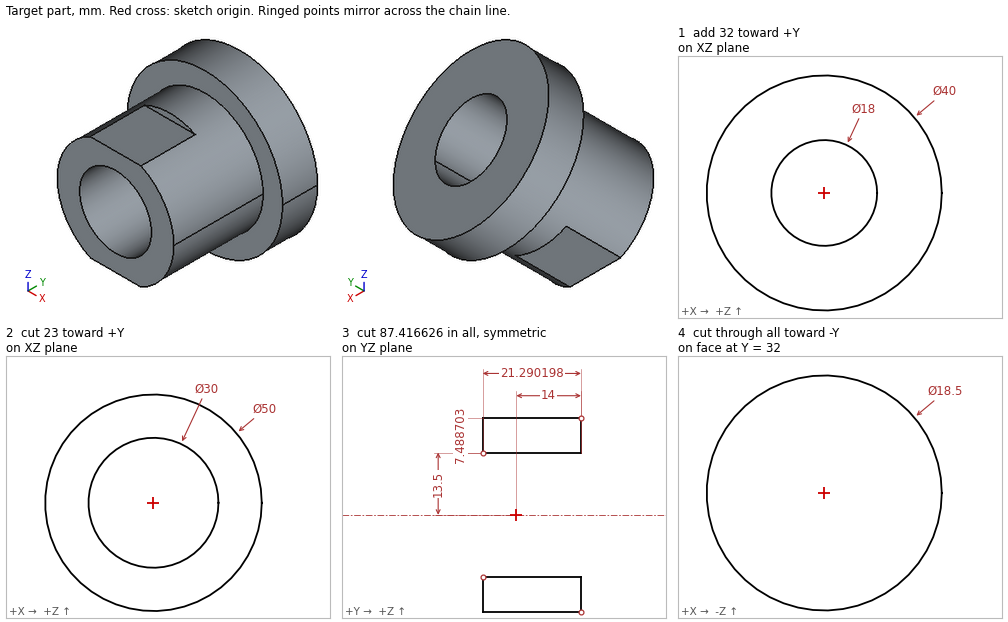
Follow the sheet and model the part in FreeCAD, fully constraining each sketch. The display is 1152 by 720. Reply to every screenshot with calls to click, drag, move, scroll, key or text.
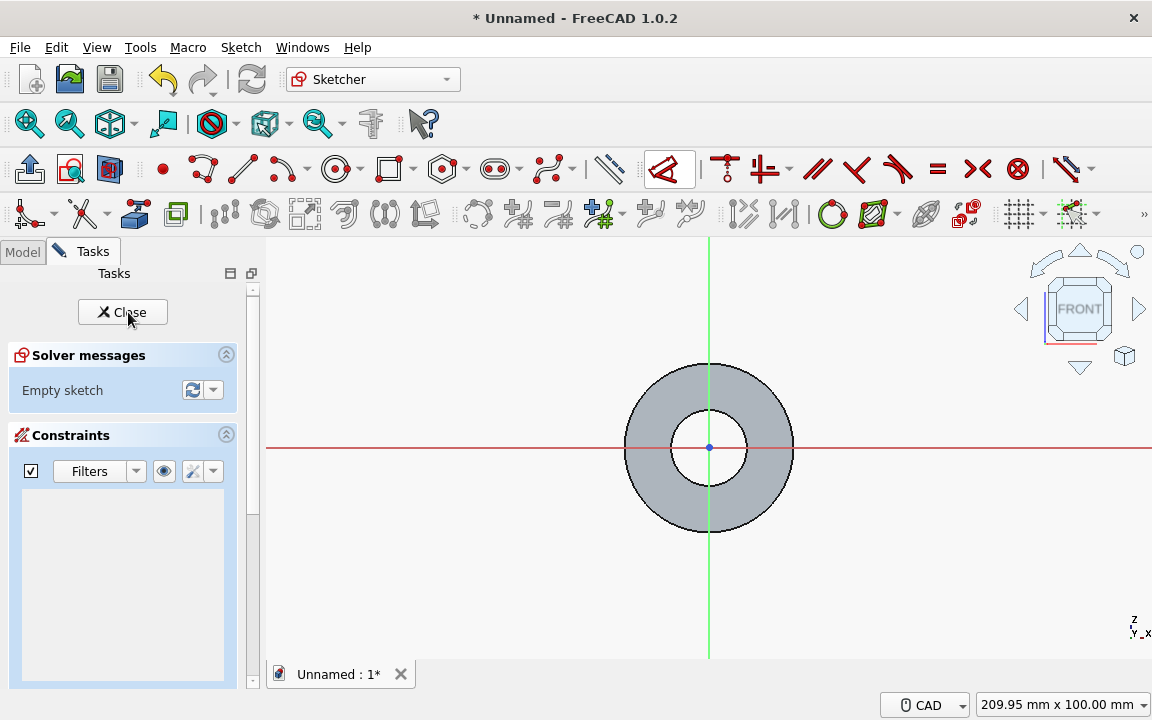
click(336, 170)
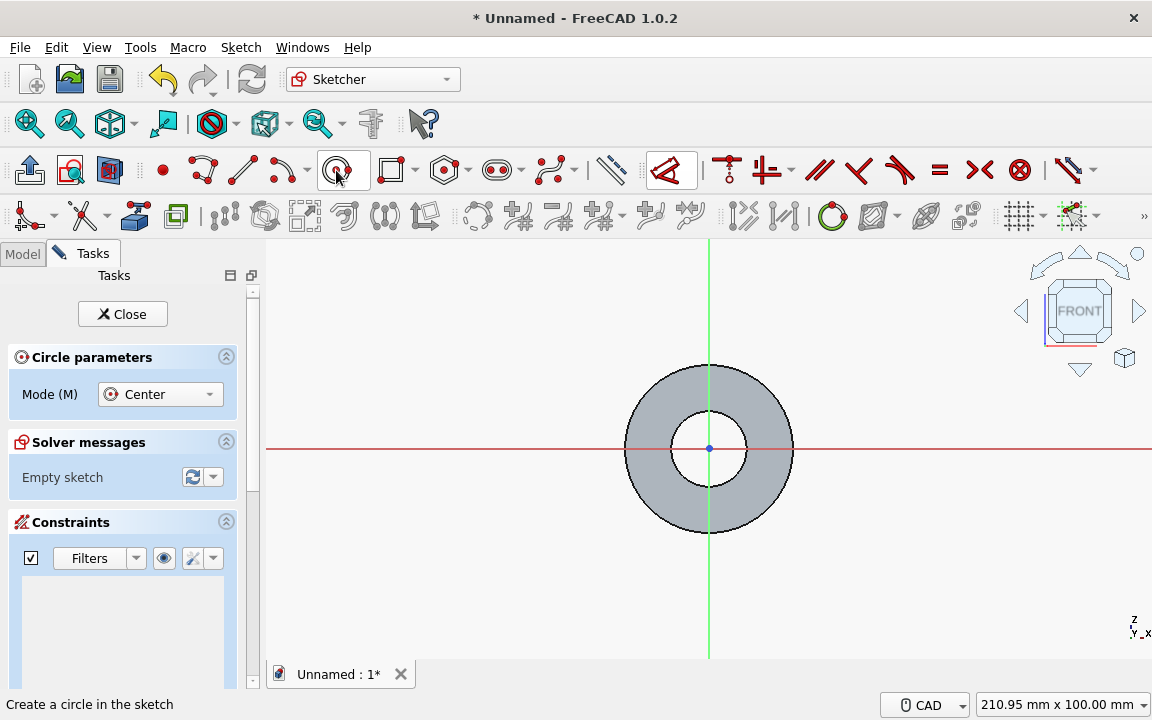
click(709, 449)
click(783, 375)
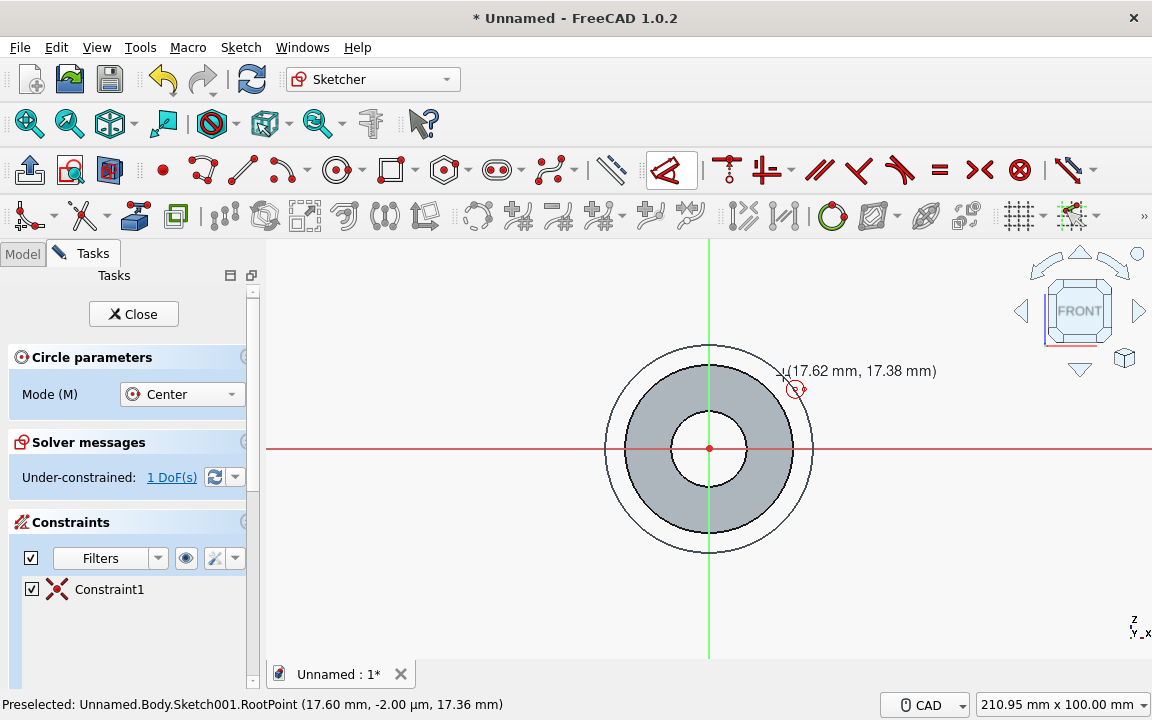
click(709, 449)
click(754, 404)
key(Escape)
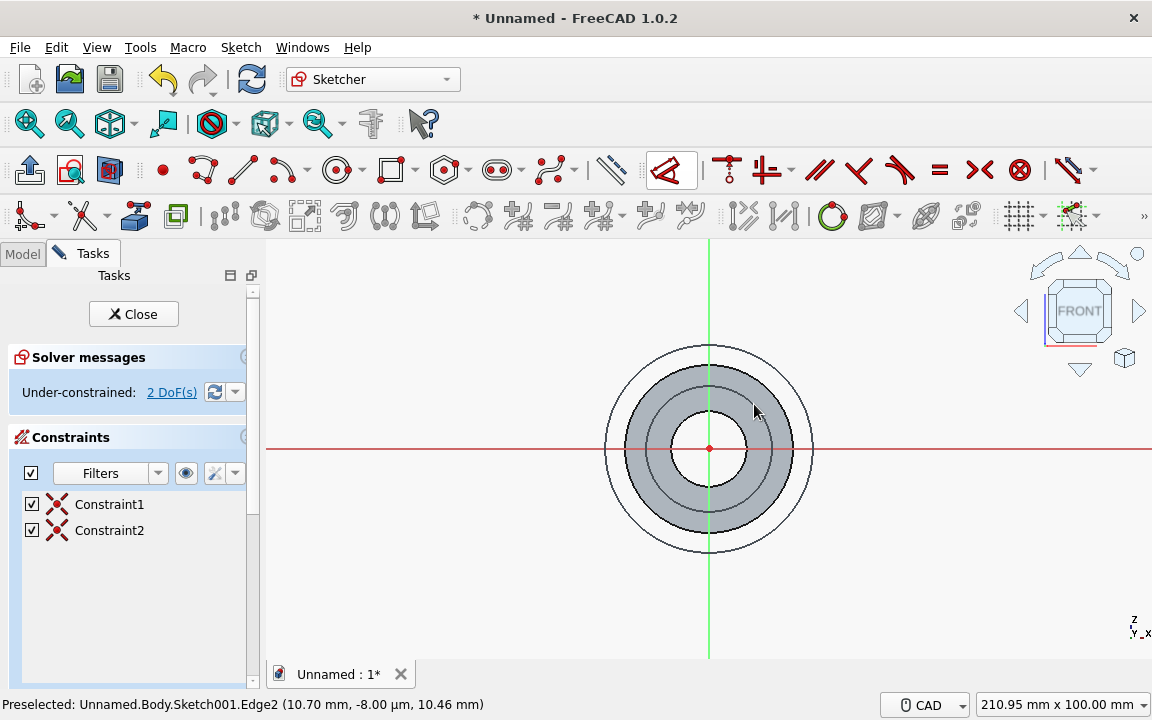
click(782, 375)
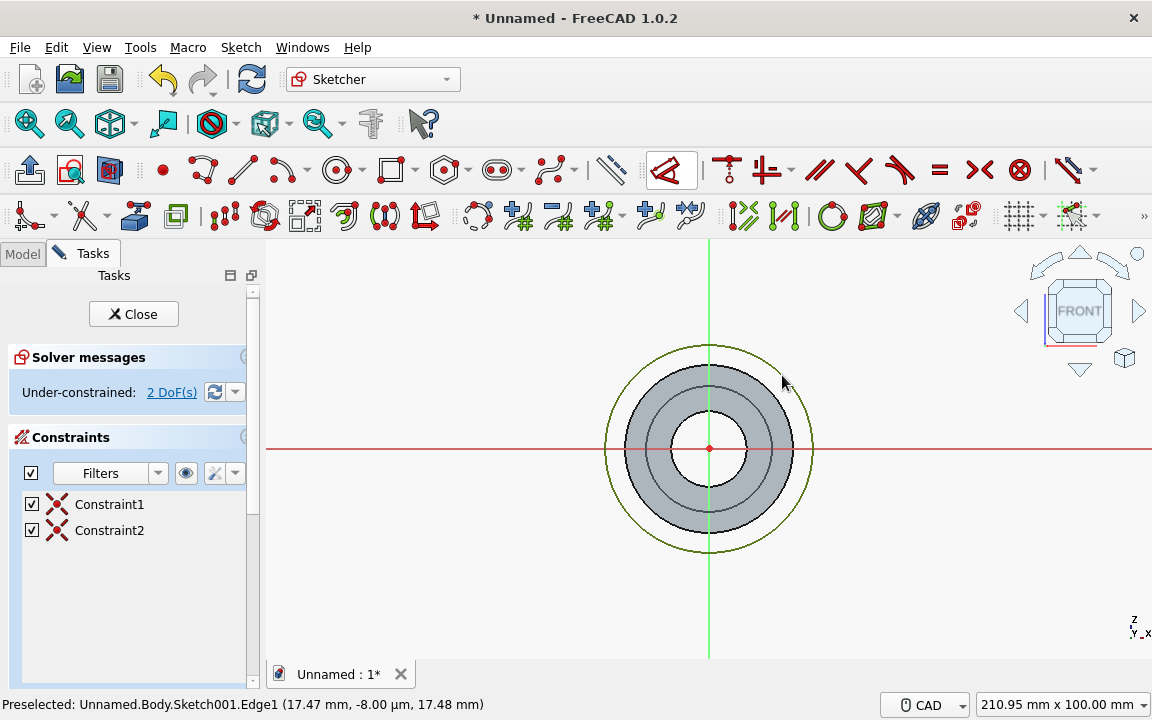
click(692, 170)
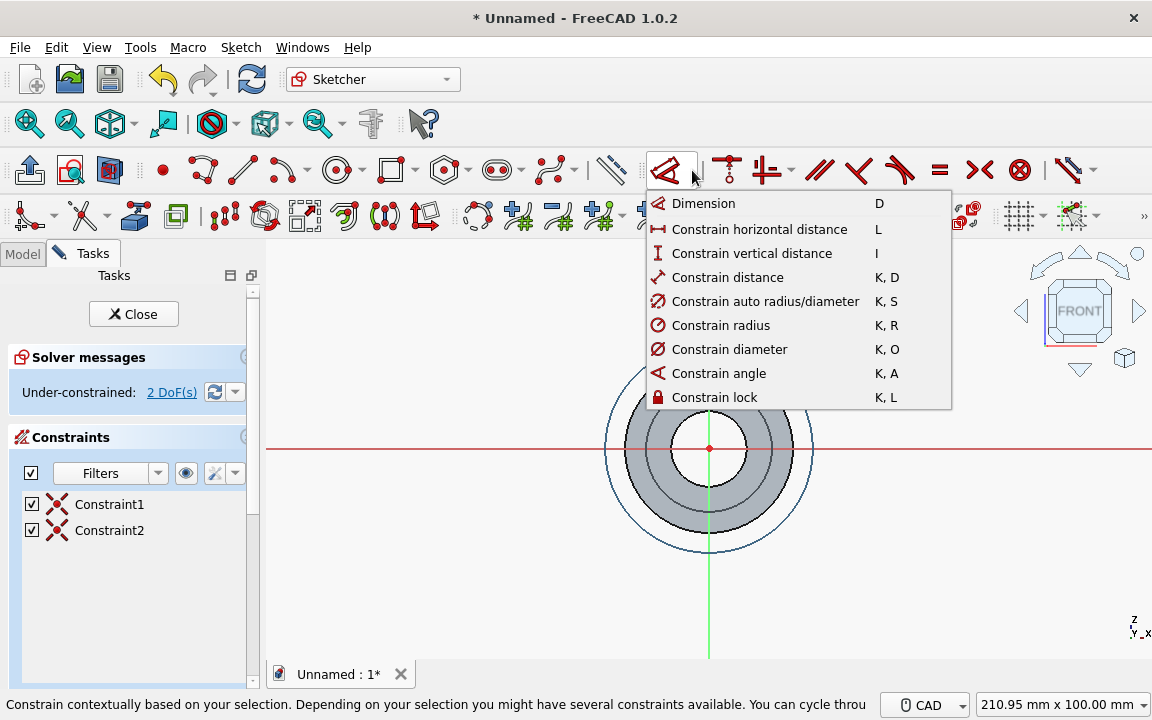
click(799, 349)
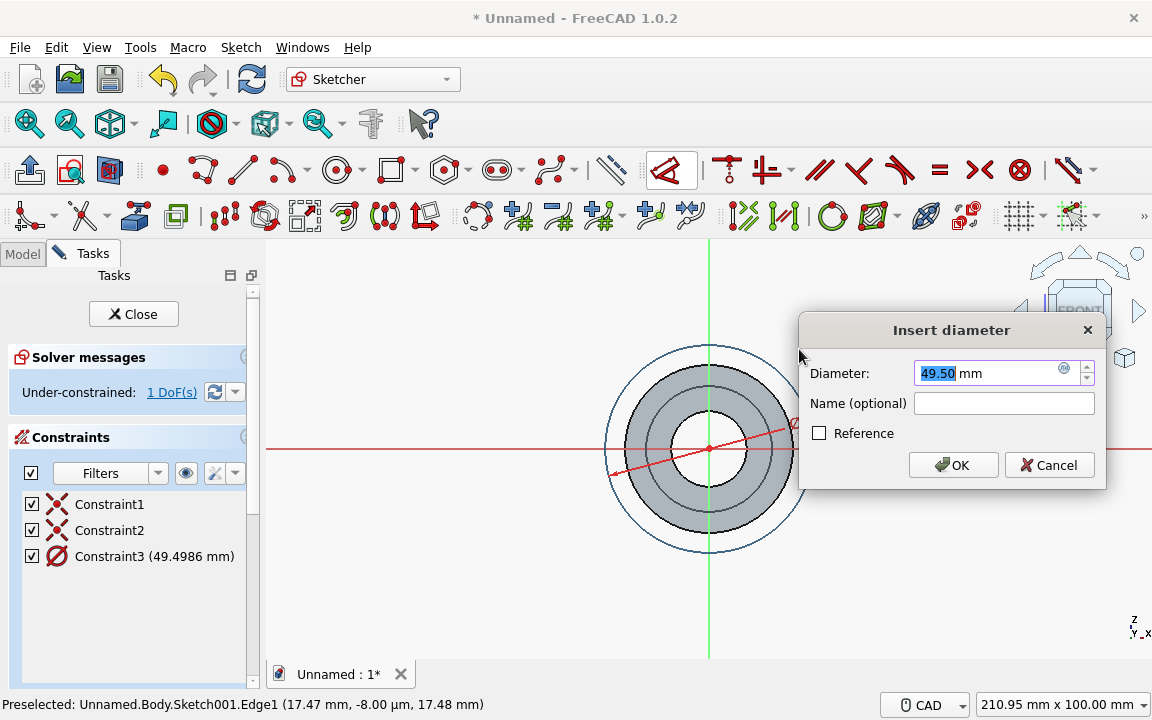
text(50)
key(Return)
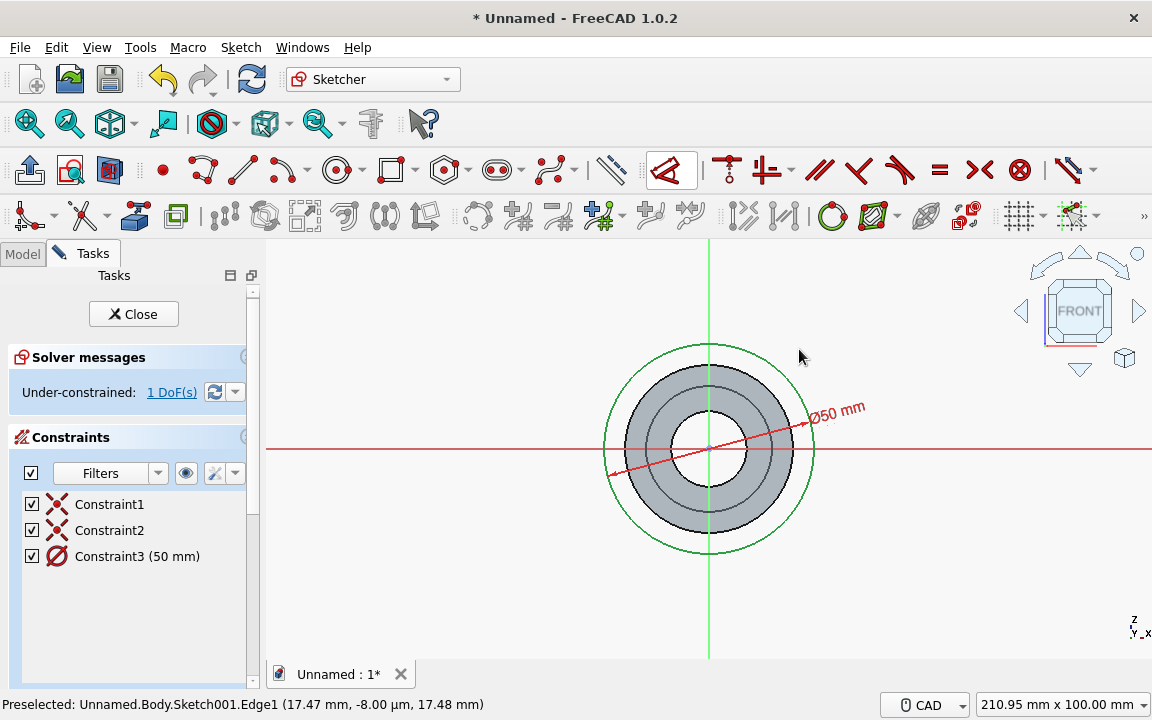
click(753, 404)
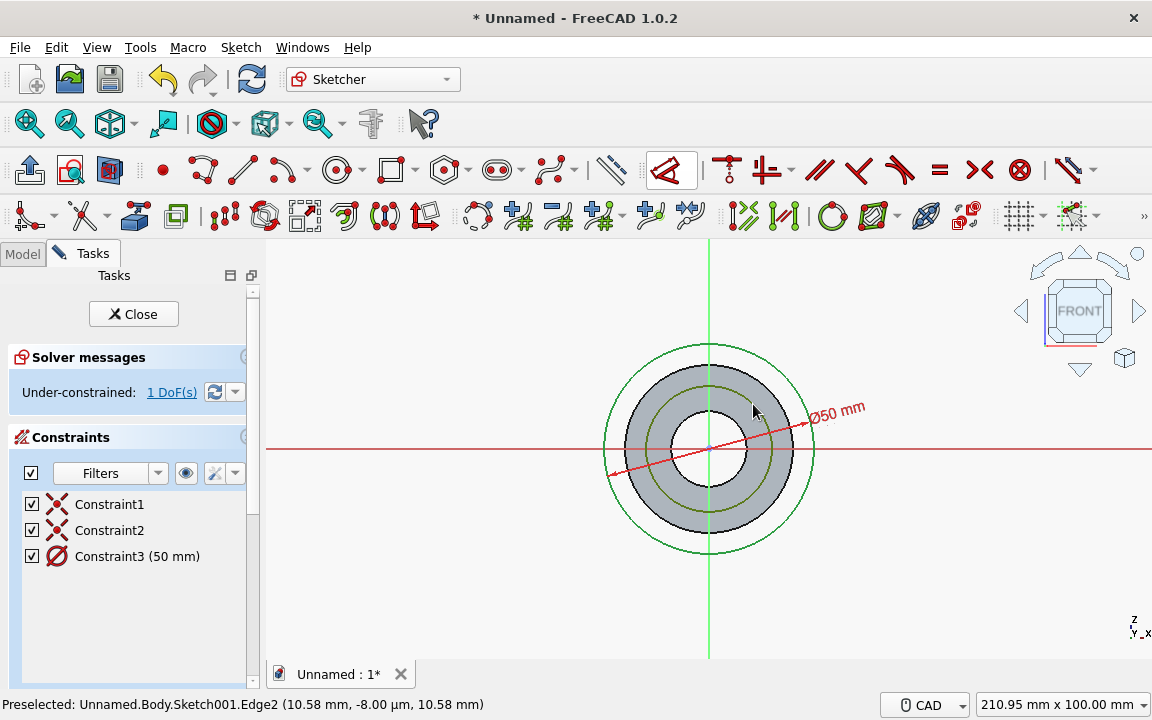
click(692, 170)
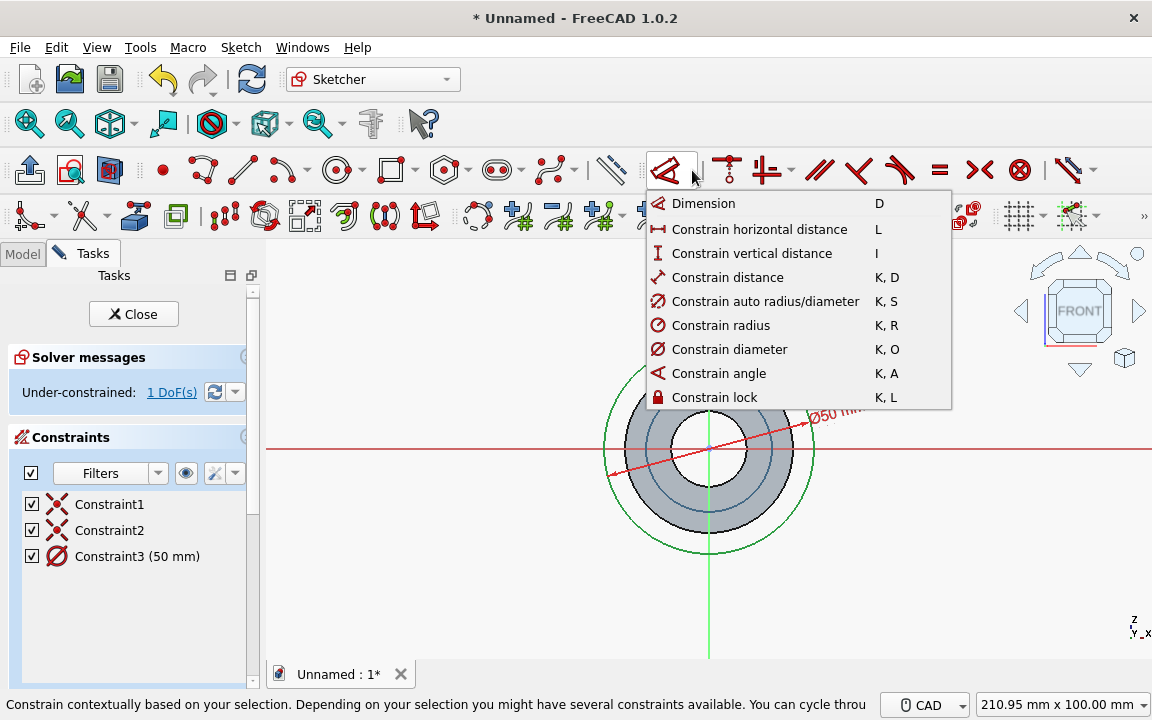
click(799, 349)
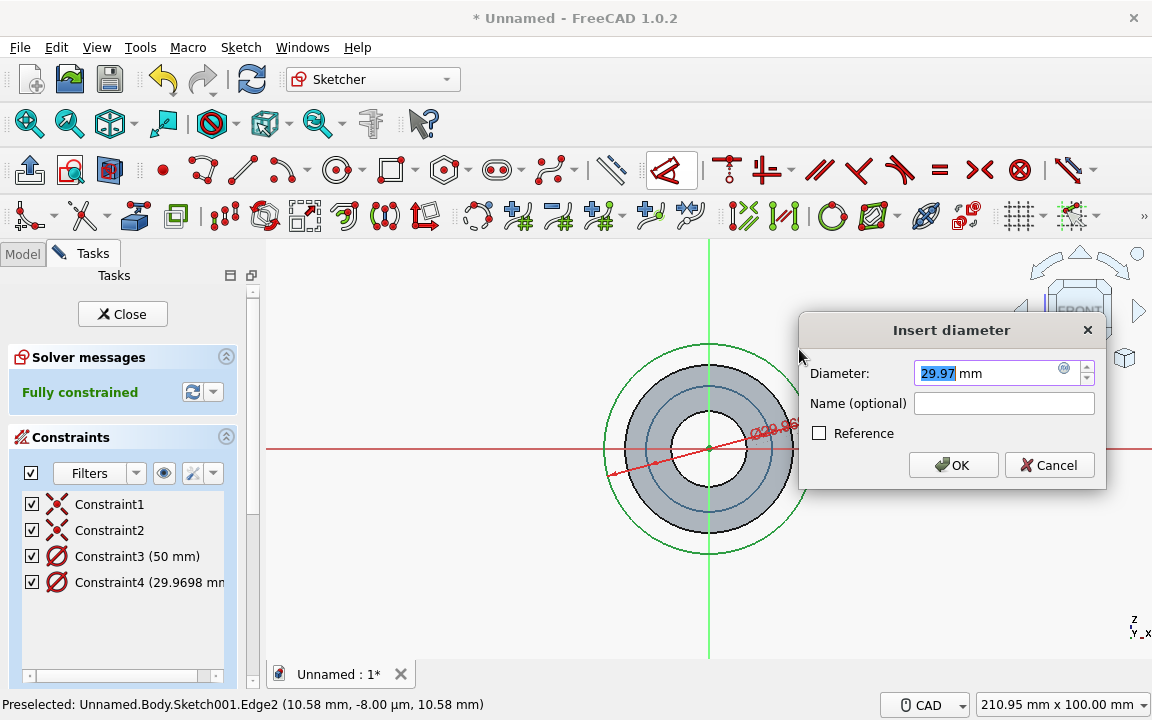
text(30)
key(Return)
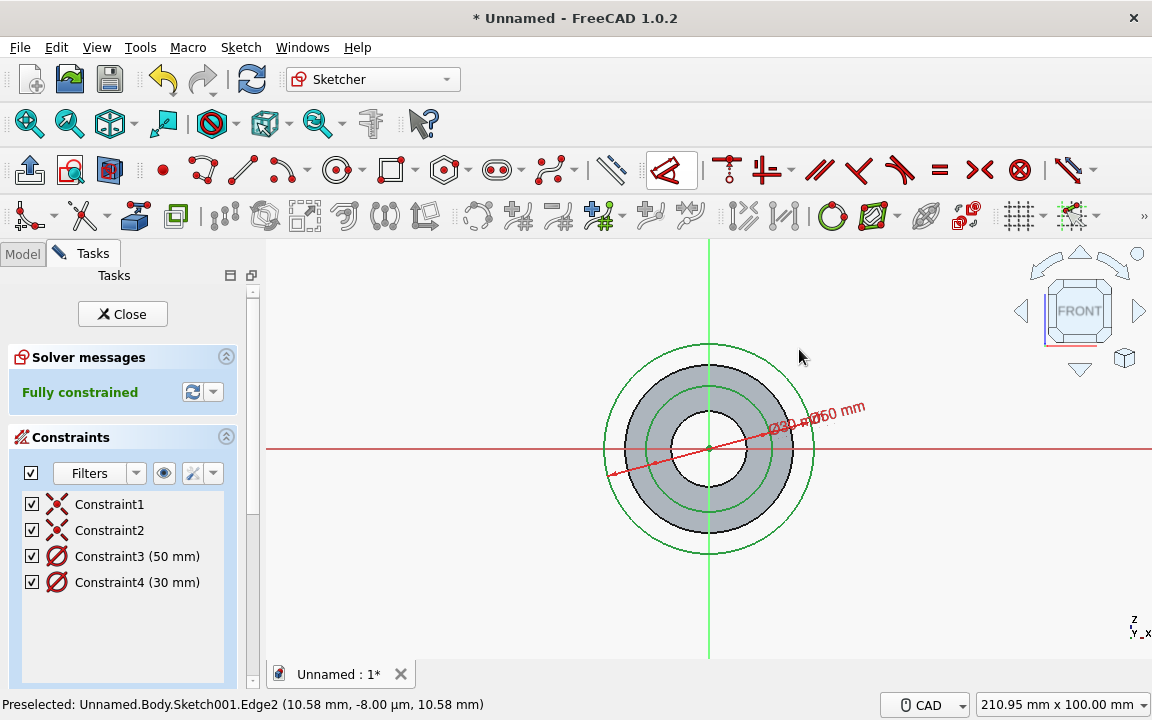
click(123, 314)